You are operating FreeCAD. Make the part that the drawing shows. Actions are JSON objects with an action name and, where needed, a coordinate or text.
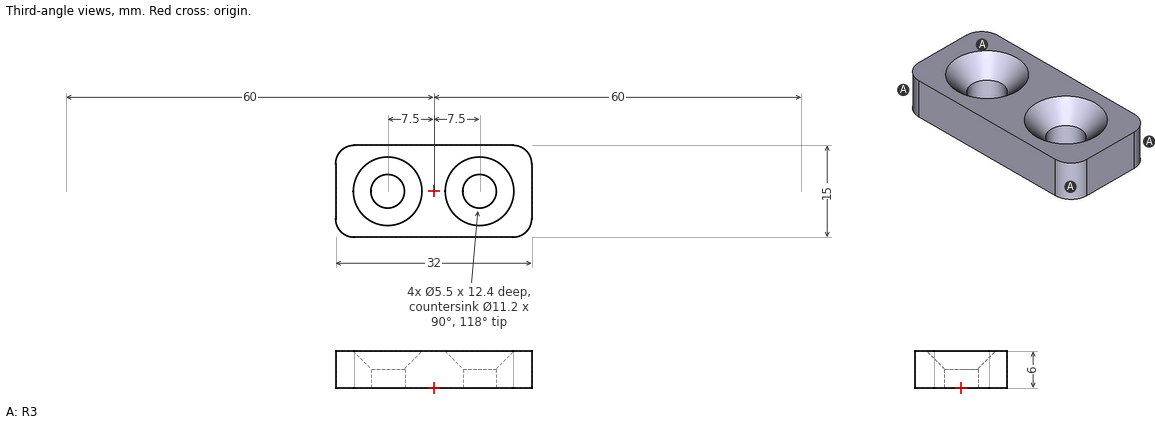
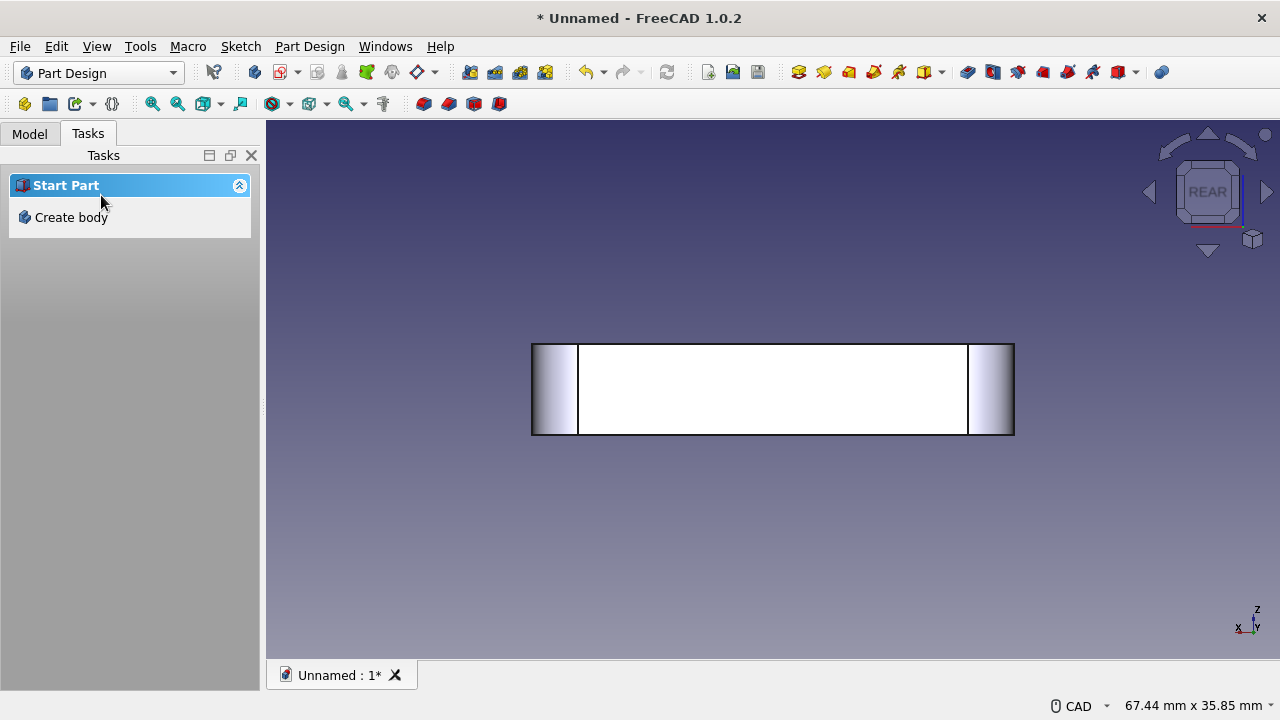
{"action": "key", "text": "0"}